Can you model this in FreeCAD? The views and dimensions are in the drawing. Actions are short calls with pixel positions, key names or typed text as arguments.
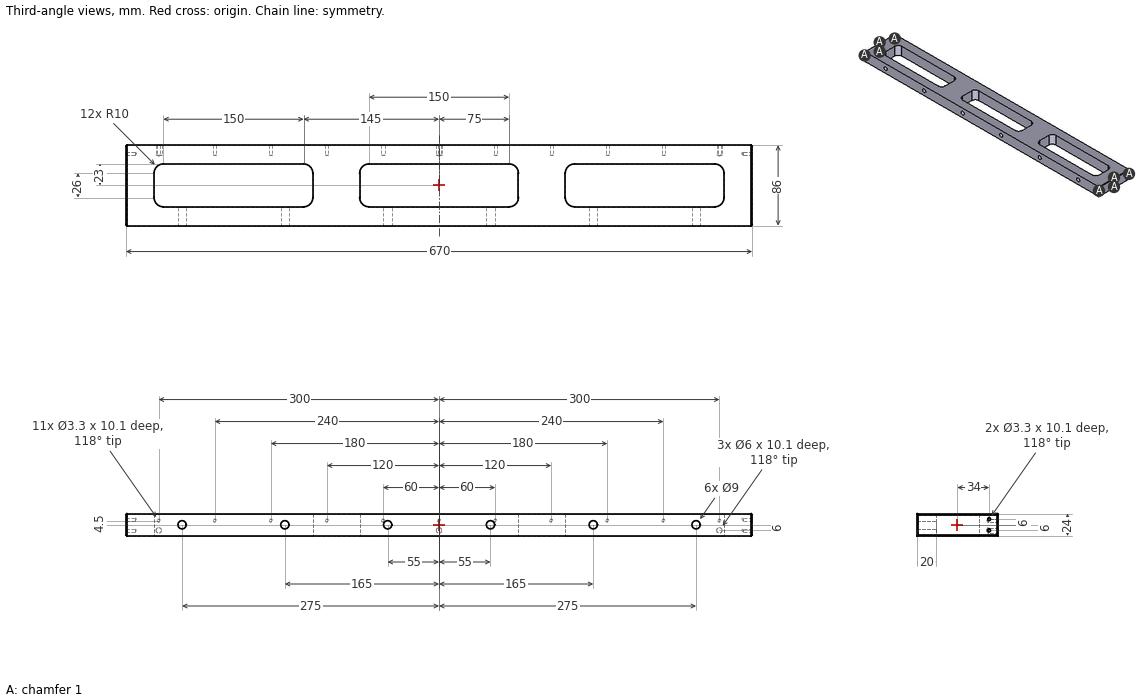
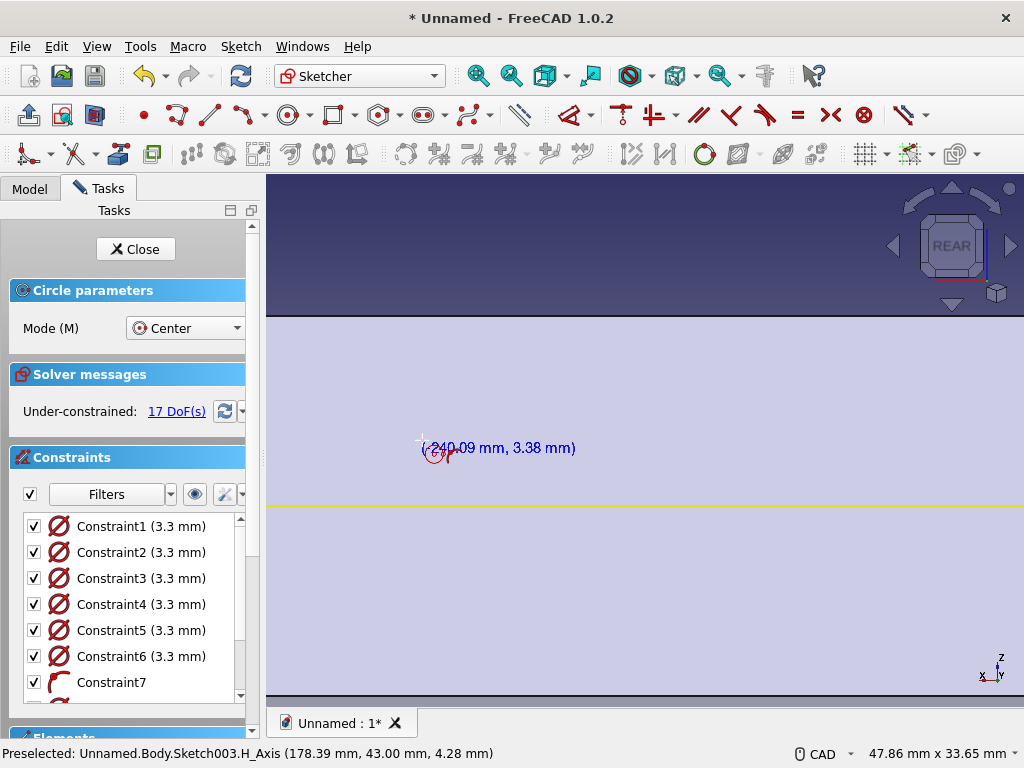
scroll(386, 440, down, 15)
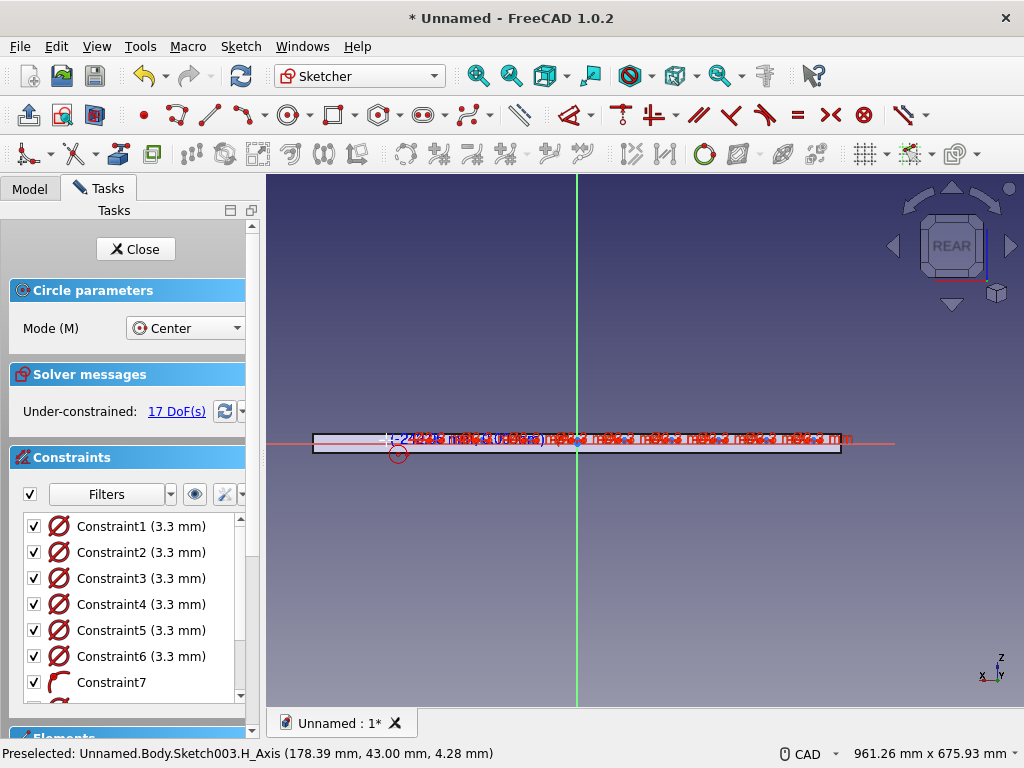
scroll(388, 440, up, 8)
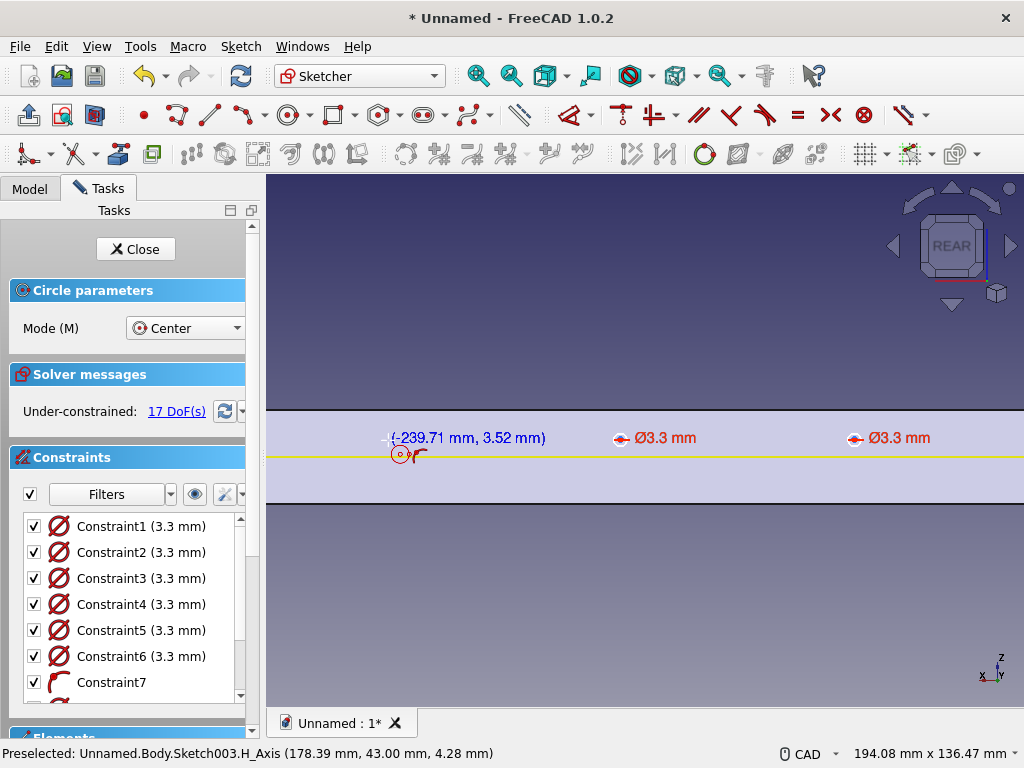
click(386, 439)
move(391, 435)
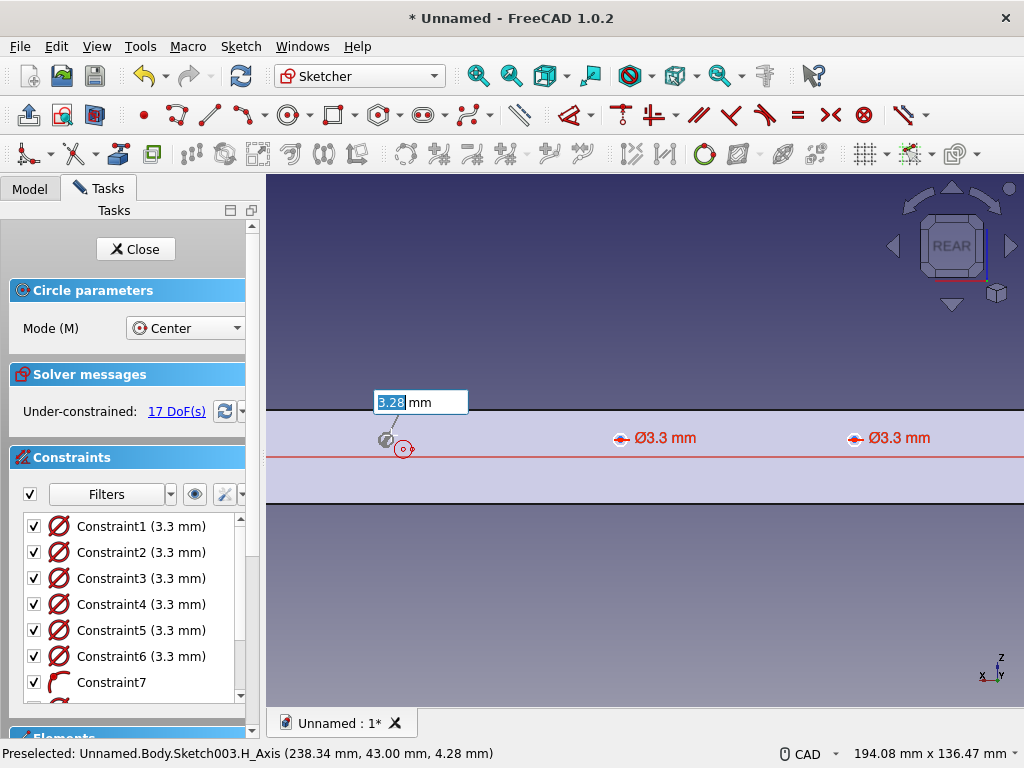
text(3.3)
key(Return)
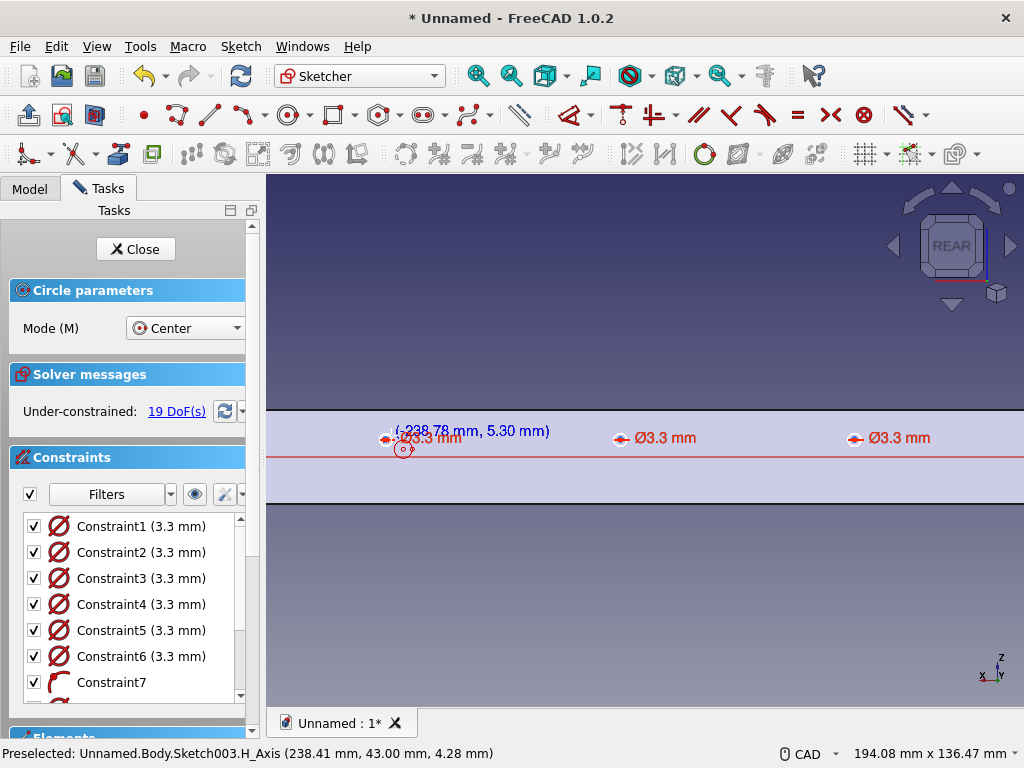
scroll(429, 440, down, 9)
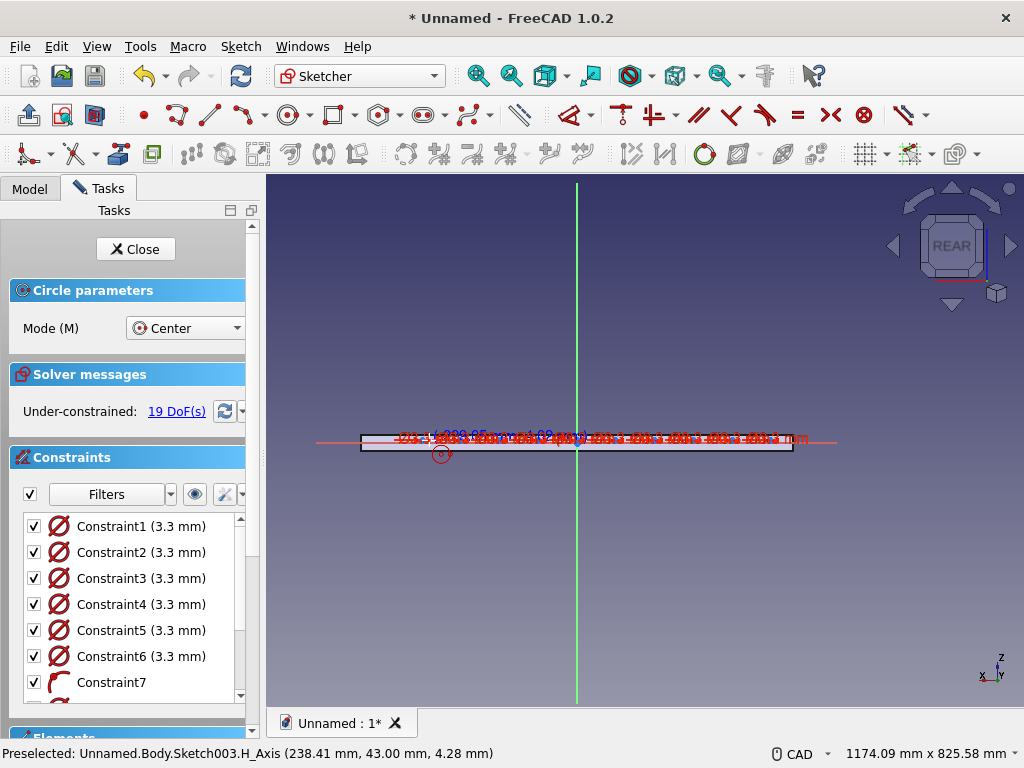
scroll(383, 440, up, 16)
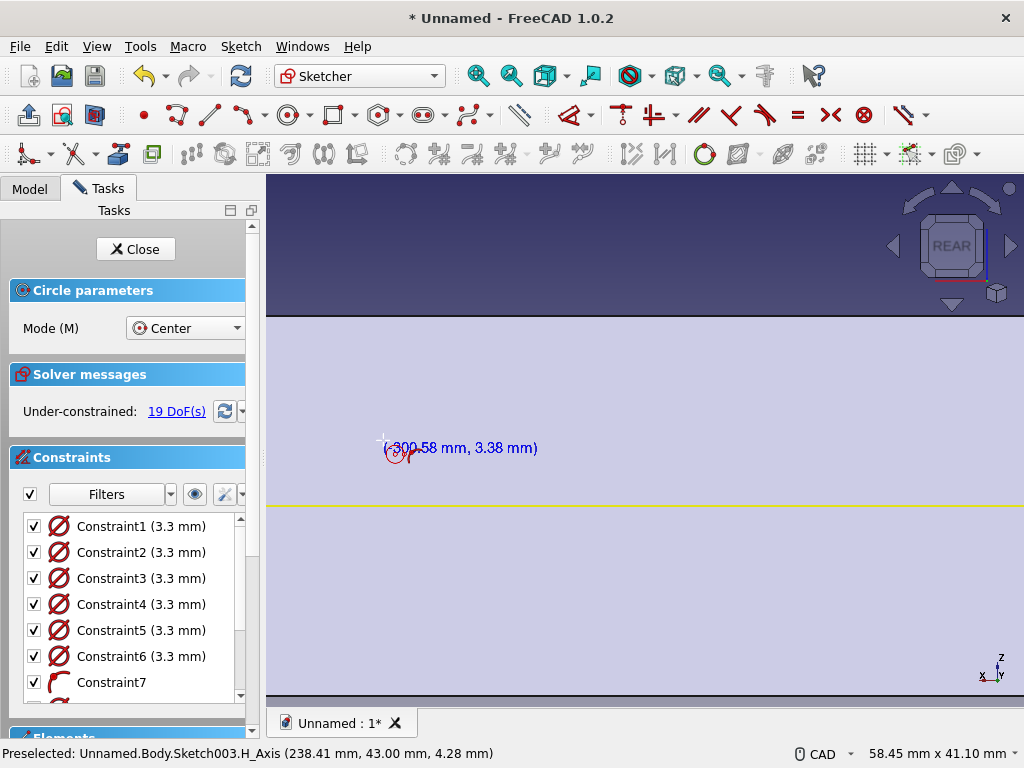
scroll(337, 440, down, 15)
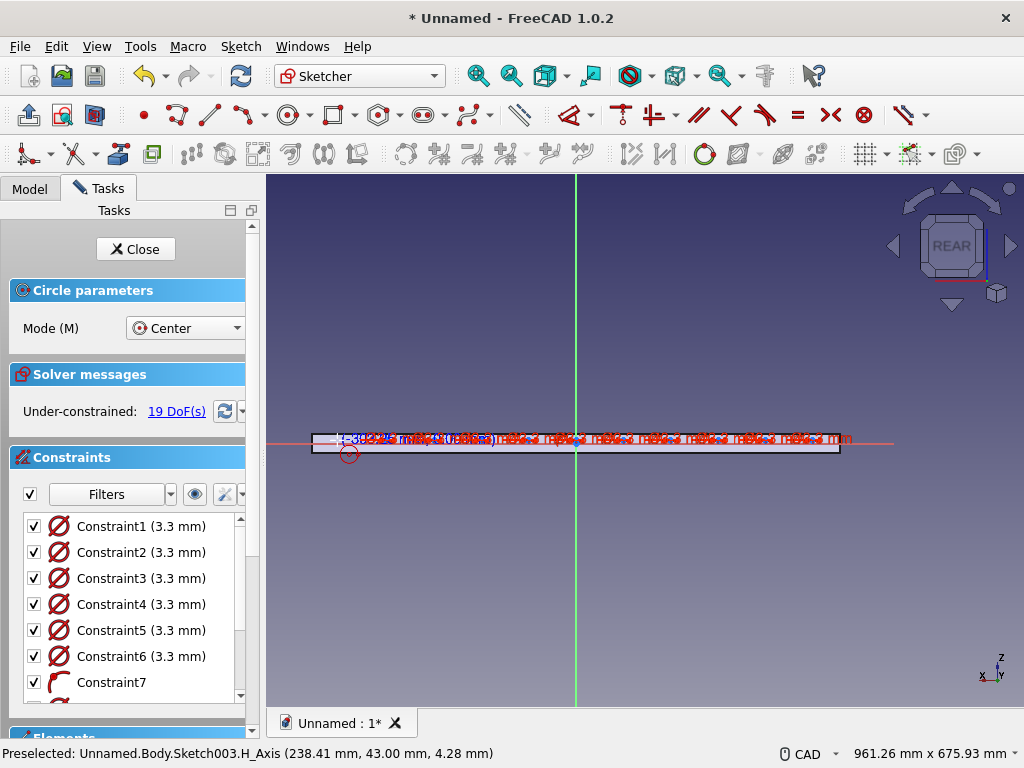
scroll(340, 440, up, 8)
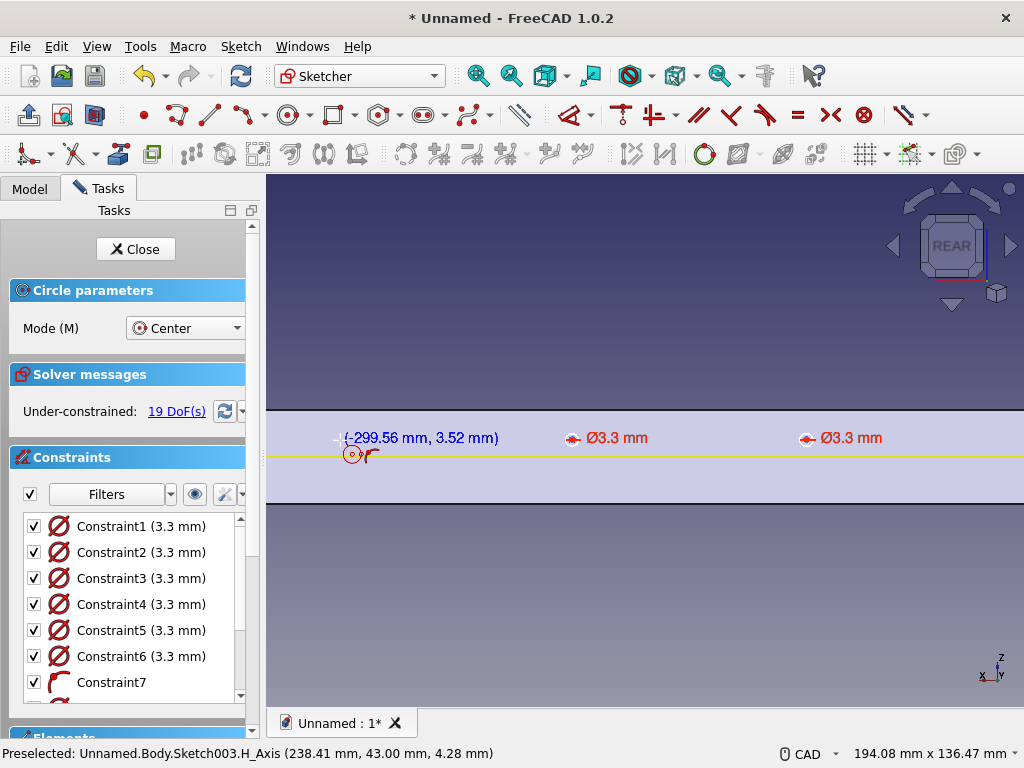
click(338, 439)
move(342, 435)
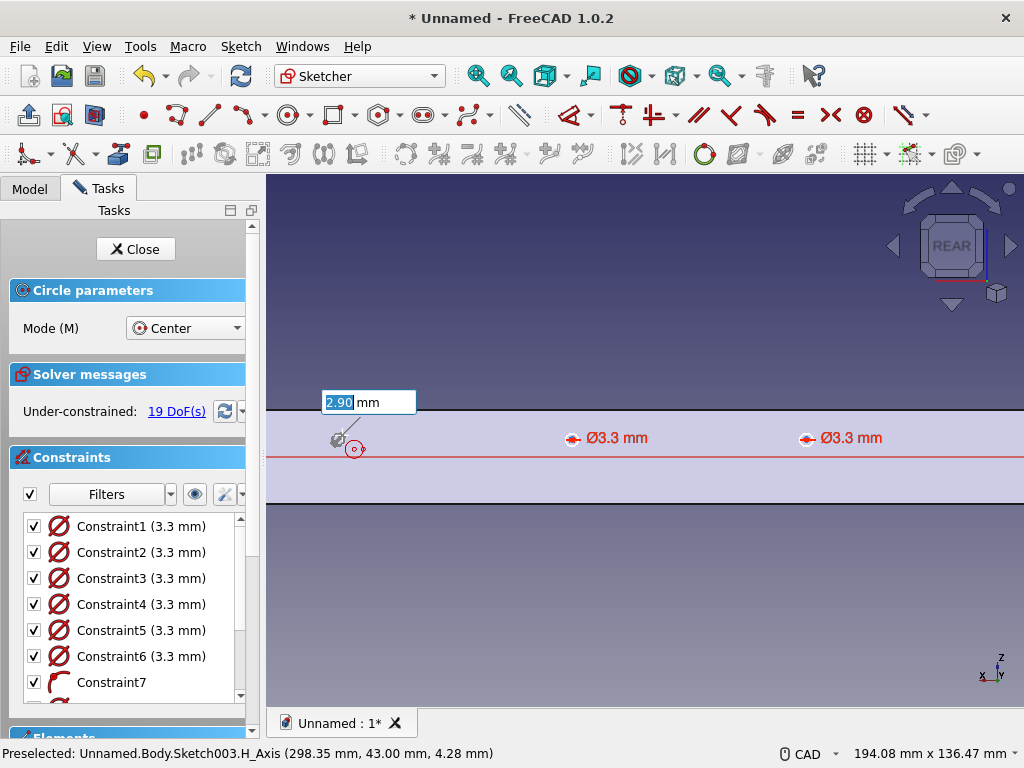
text(3.3)
key(Return)
key(Escape)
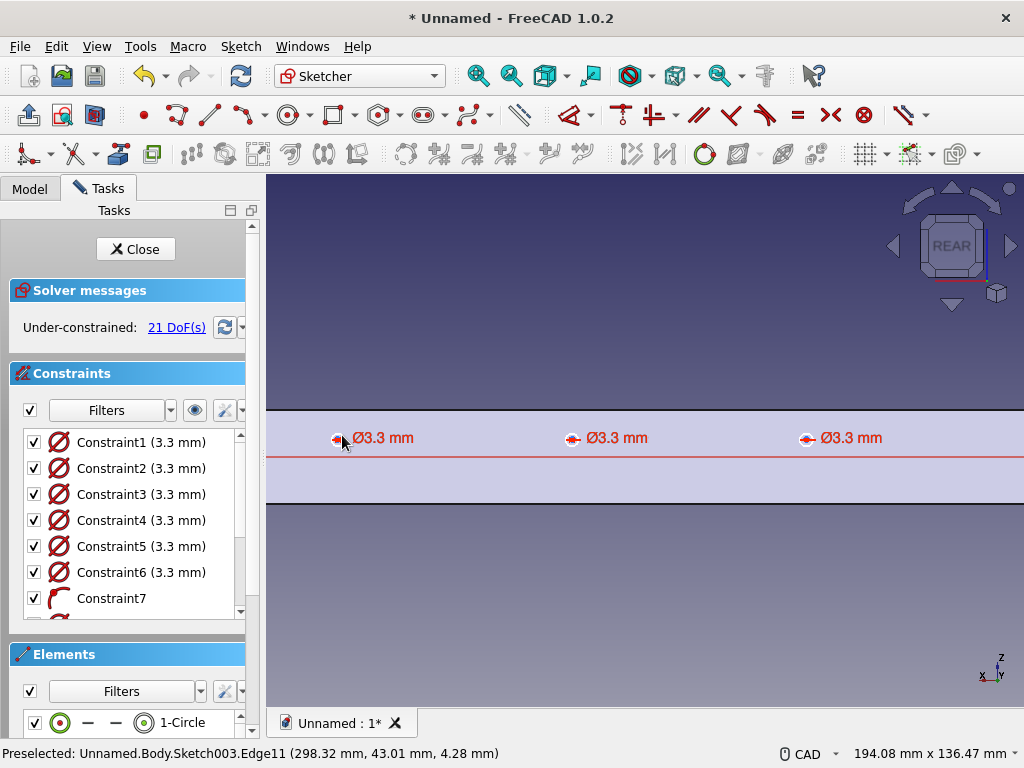
scroll(392, 440, down, 9)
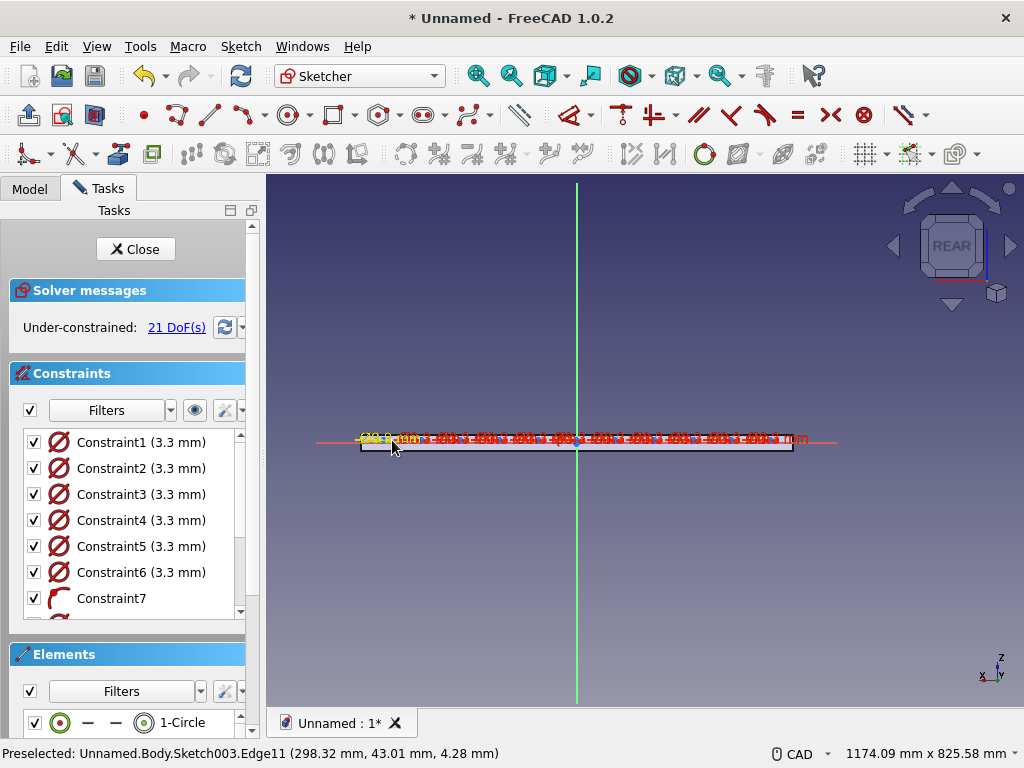
click(771, 440)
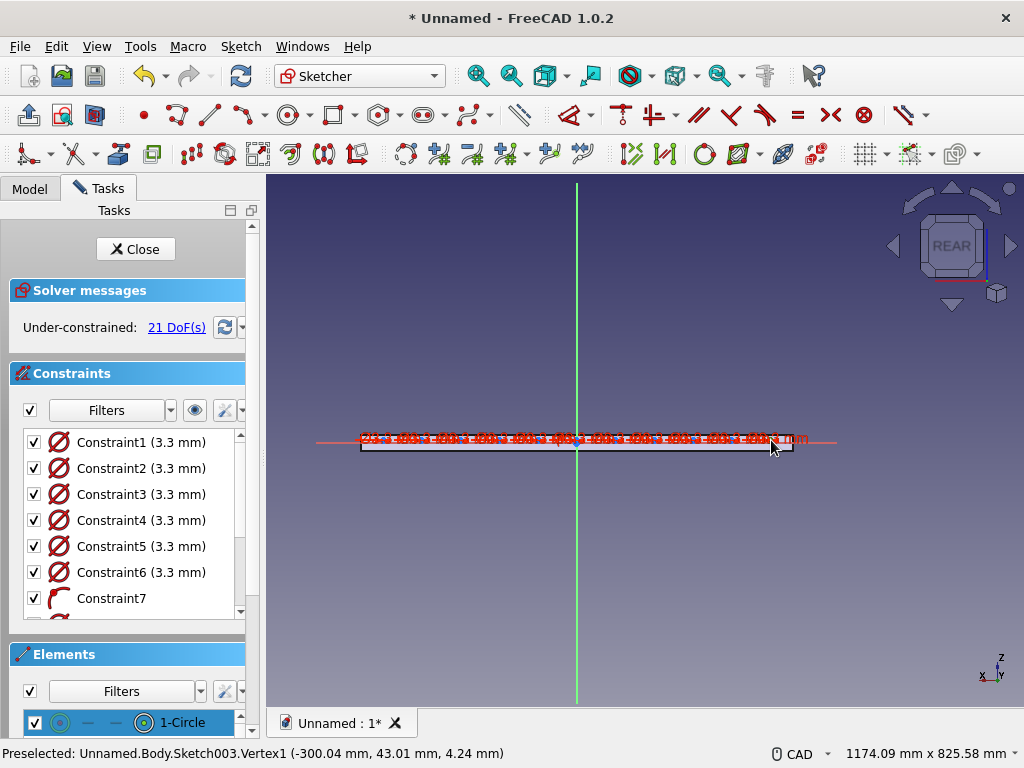
click(732, 440)